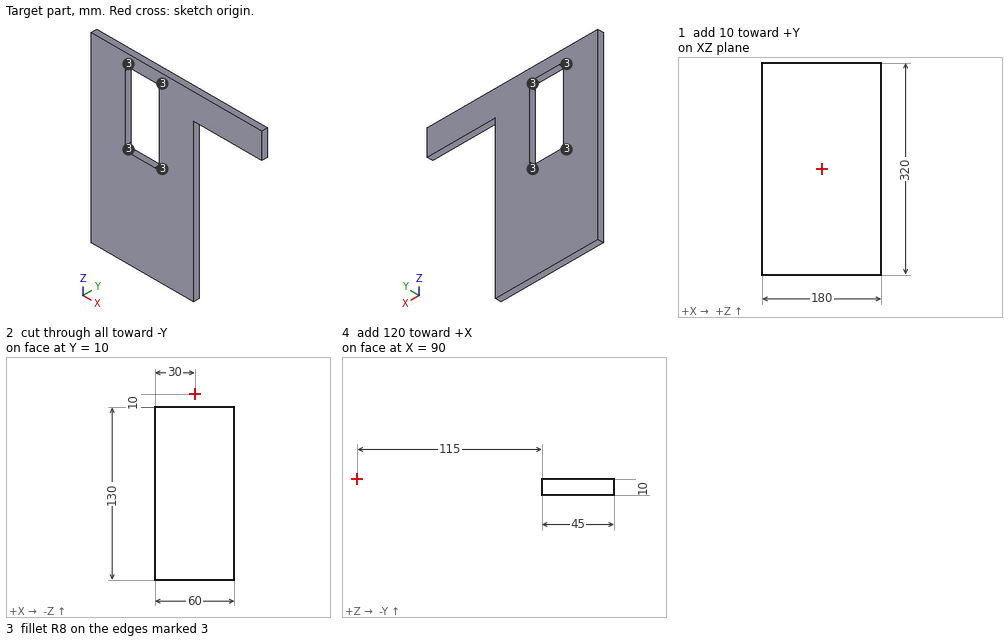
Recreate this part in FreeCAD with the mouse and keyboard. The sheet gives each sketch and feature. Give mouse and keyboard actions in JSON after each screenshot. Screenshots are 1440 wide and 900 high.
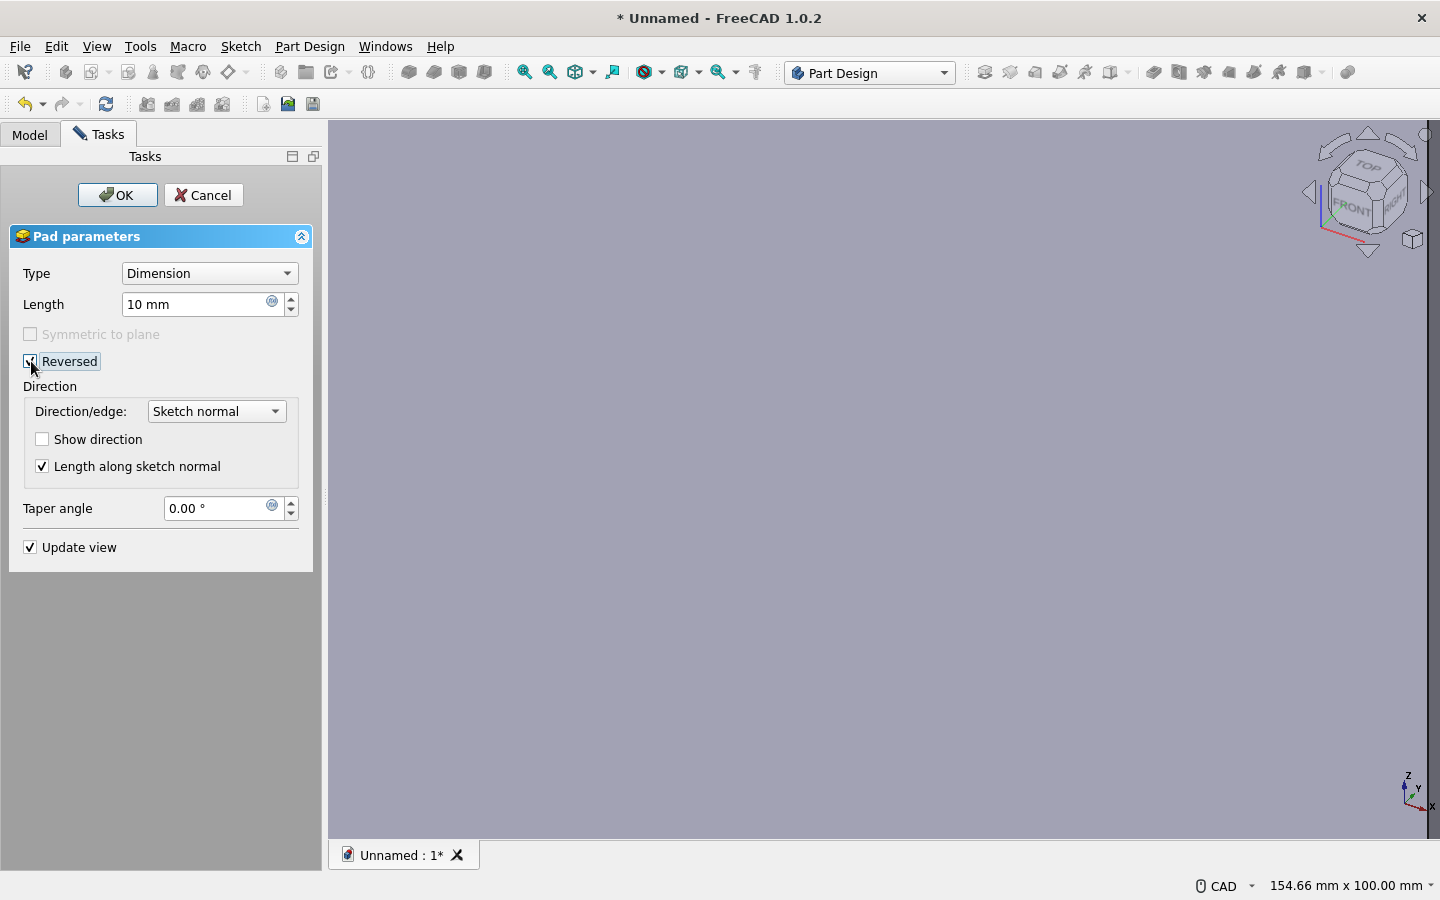
{"action": "left_click", "coordinate": [118, 195]}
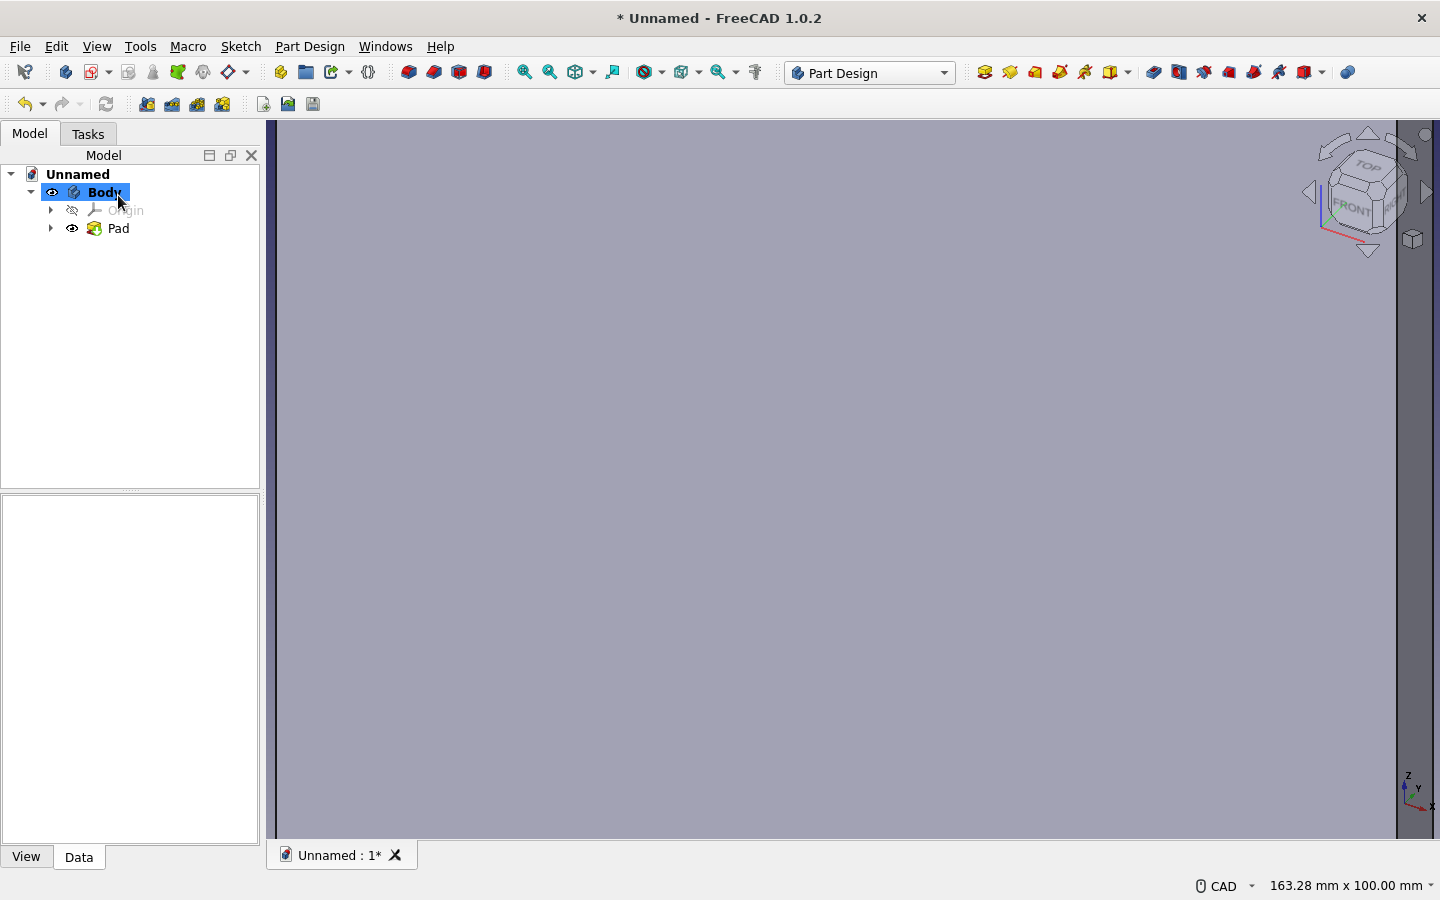
{"action": "key", "text": "v f"}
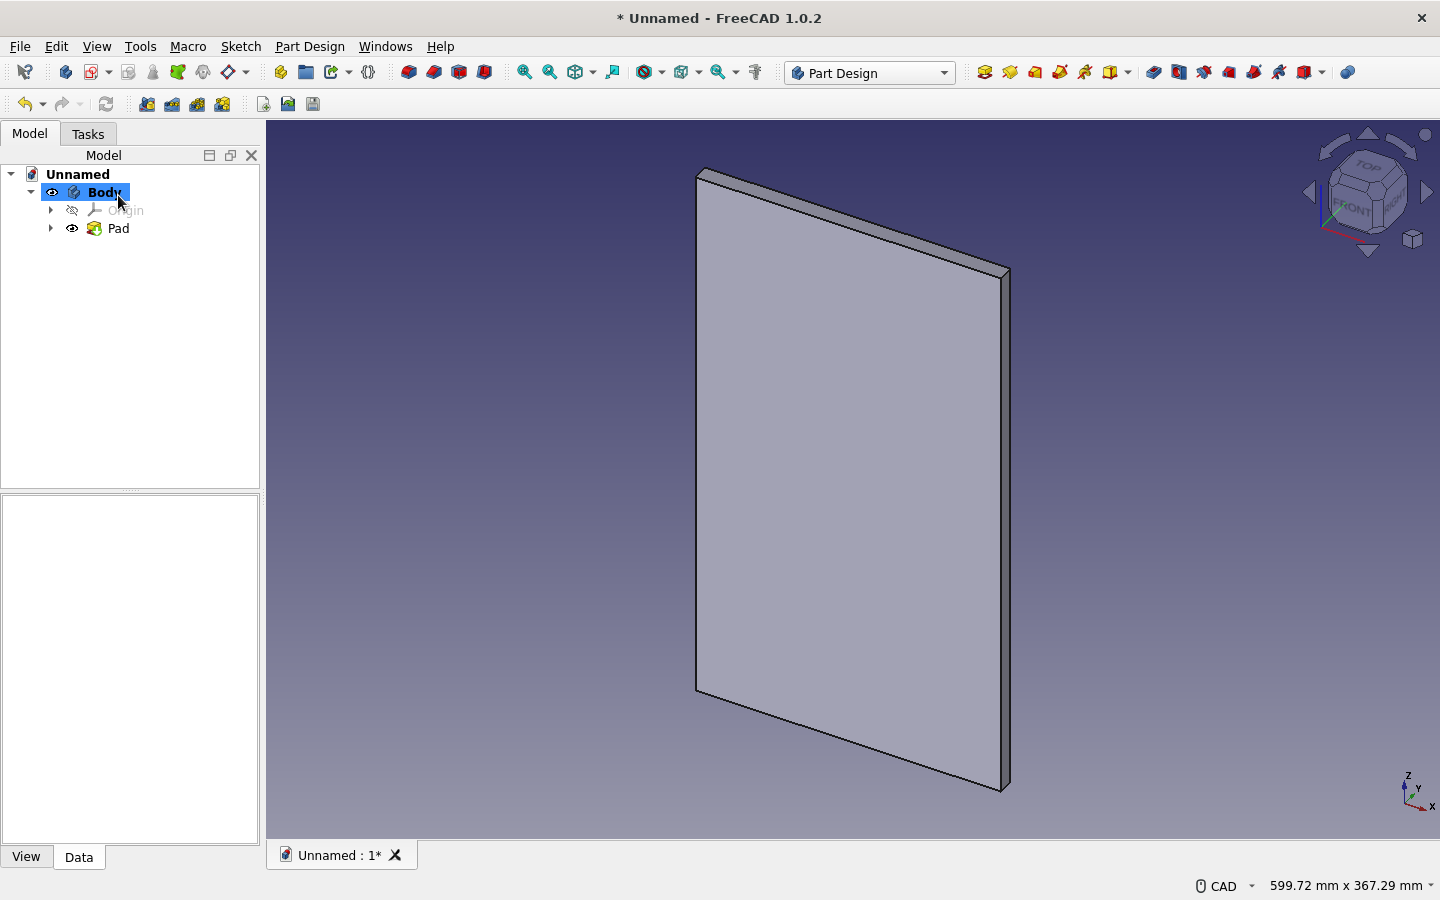
{"action": "key", "text": "4"}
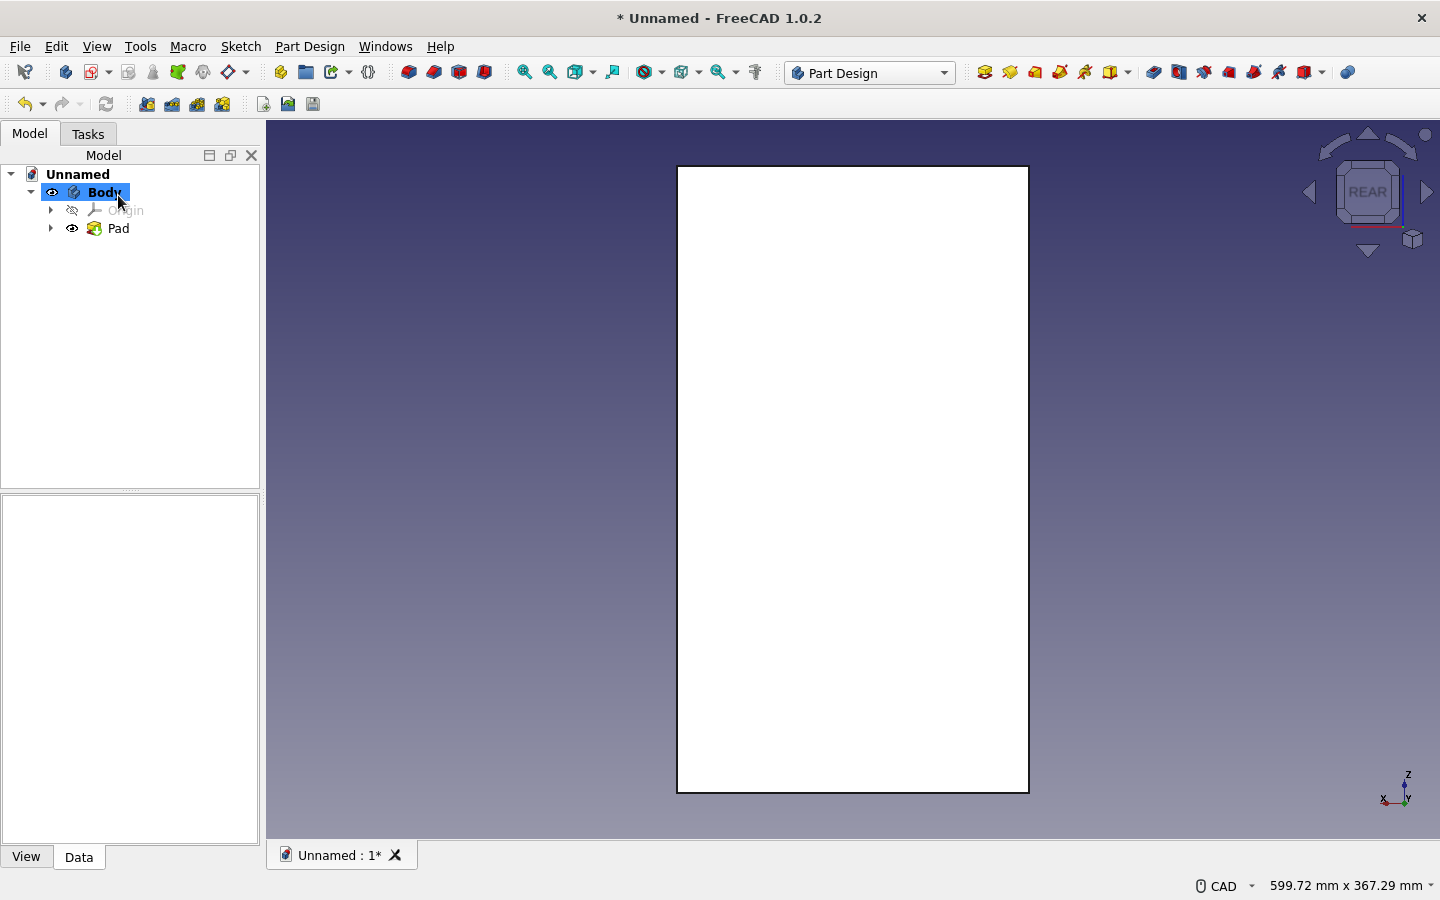
{"action": "left_click", "coordinate": [853, 389]}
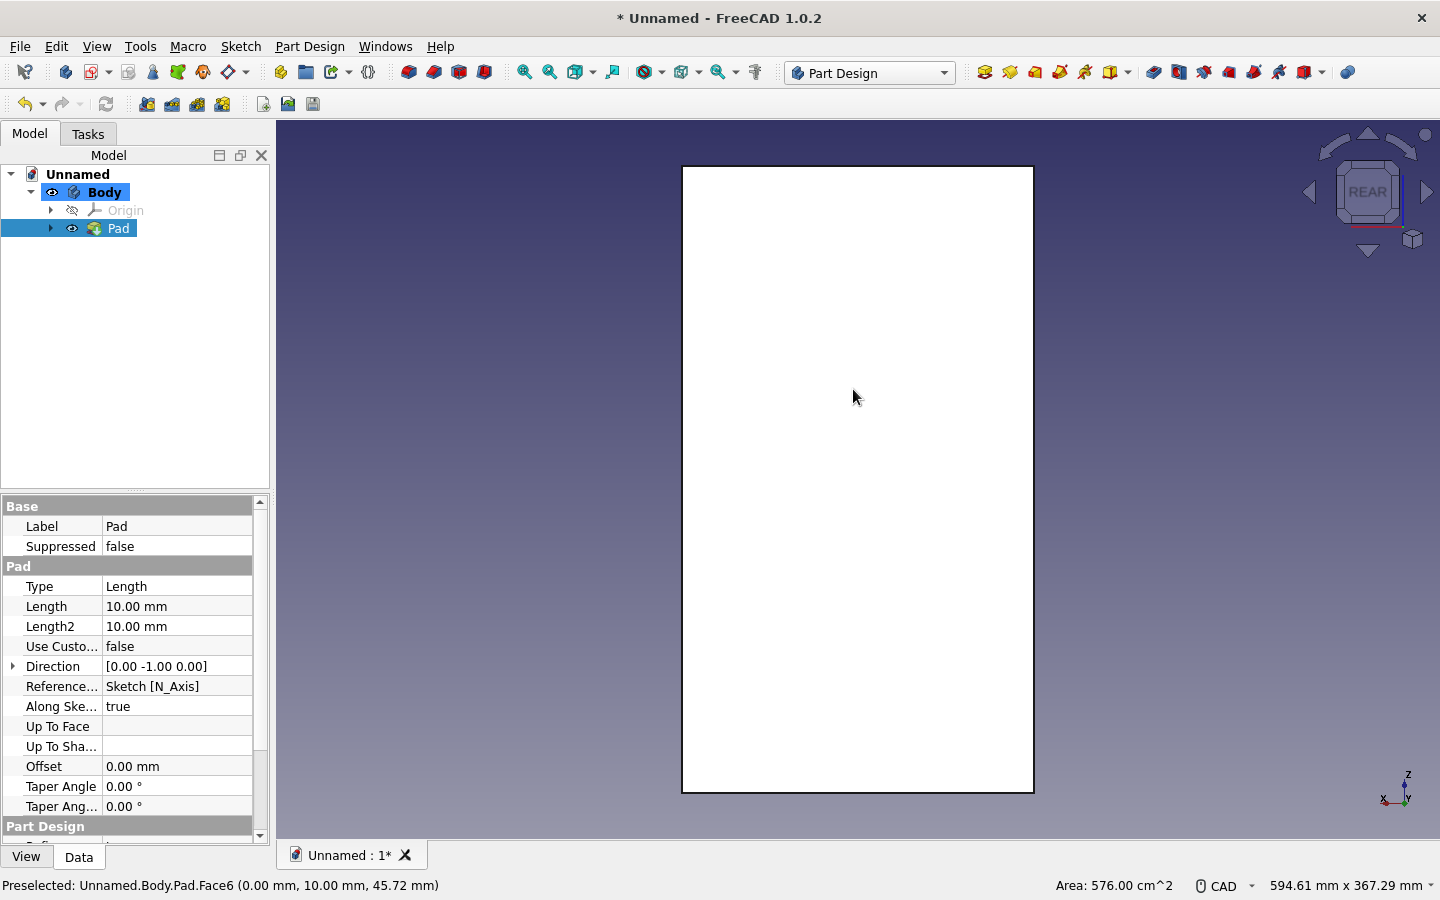
{"action": "left_click", "coordinate": [90, 72]}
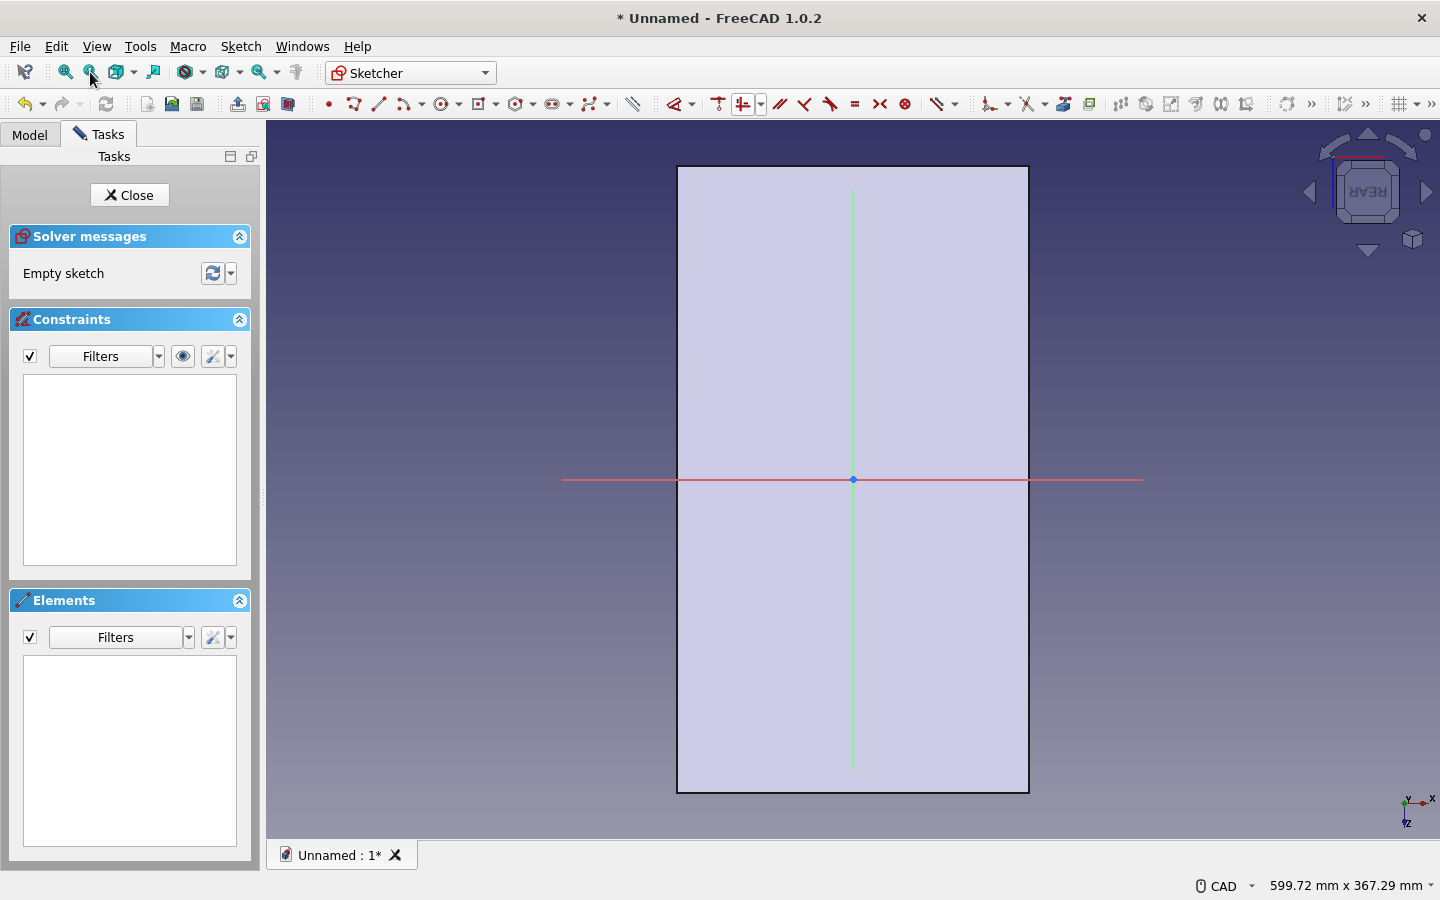
{"action": "scroll", "coordinate": [936, 783], "scroll_direction": "up", "scroll_amount": 3}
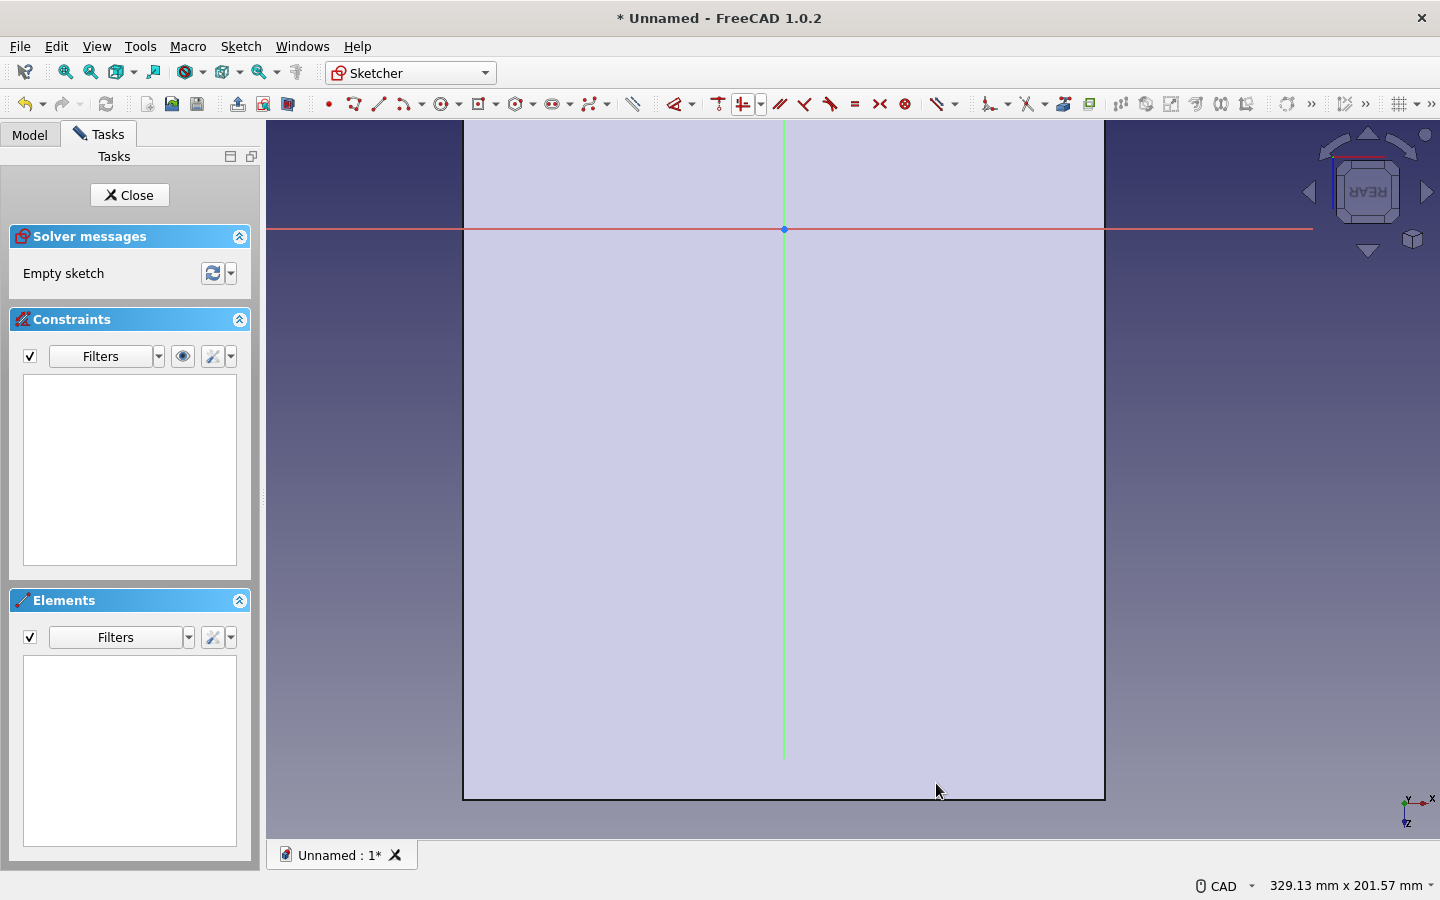
{"action": "key", "text": "g r"}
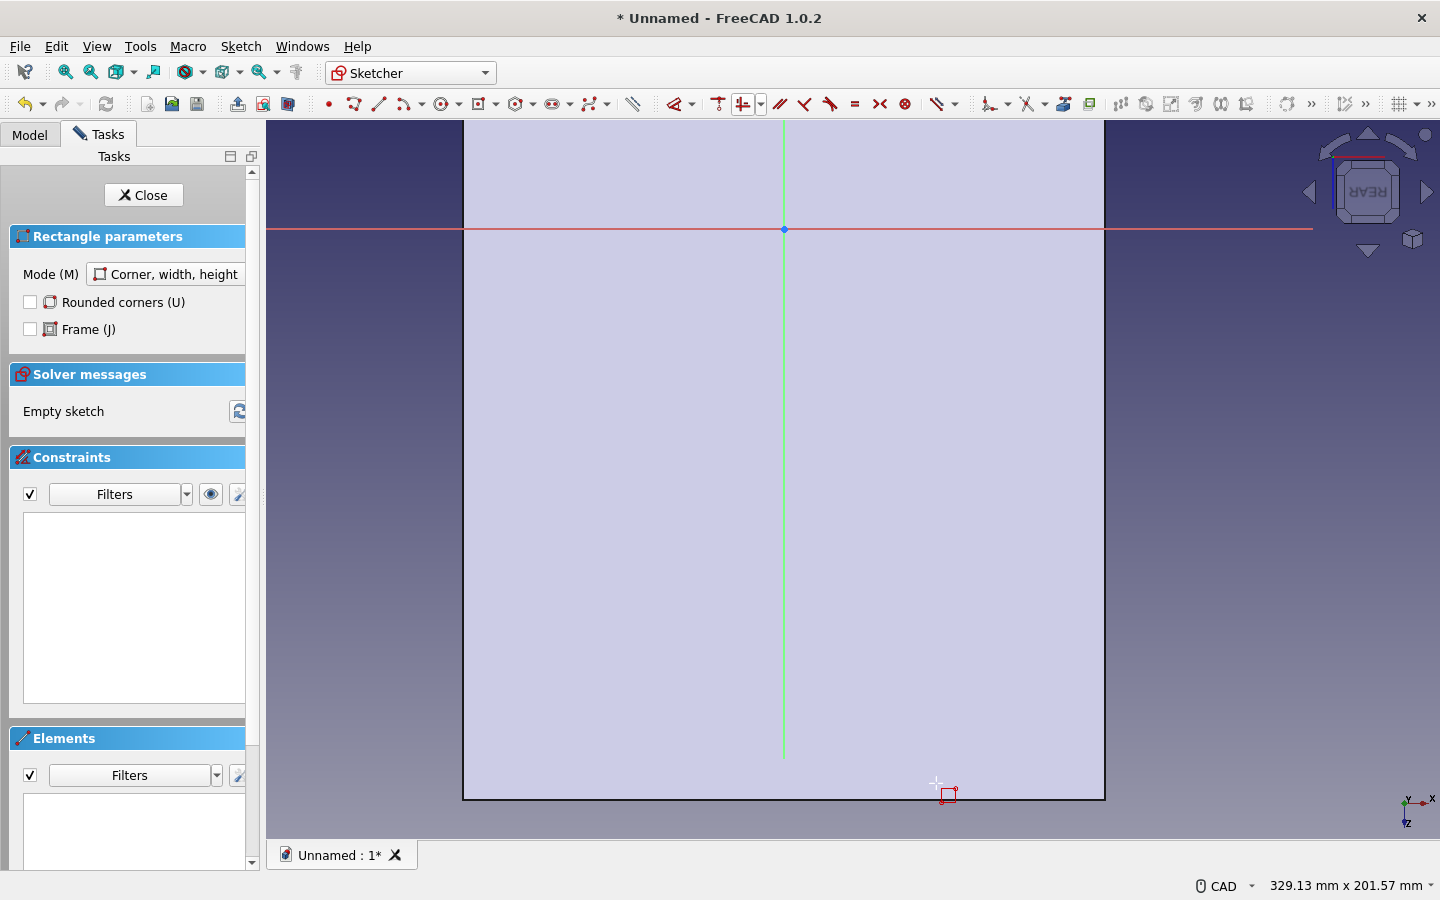
{"action": "left_click", "coordinate": [677, 265]}
{"action": "left_click", "coordinate": [891, 729]}
{"action": "key", "text": "Escape"}